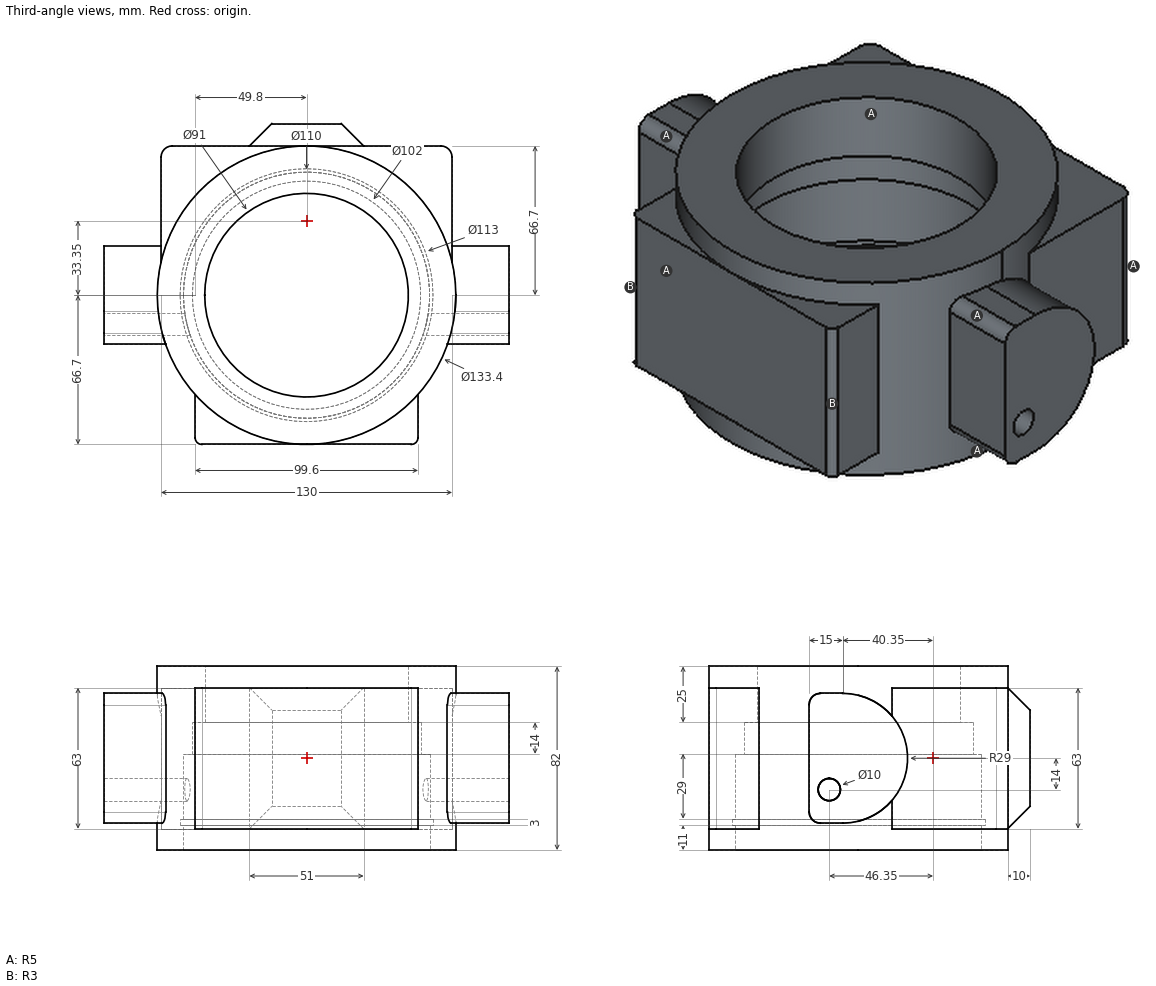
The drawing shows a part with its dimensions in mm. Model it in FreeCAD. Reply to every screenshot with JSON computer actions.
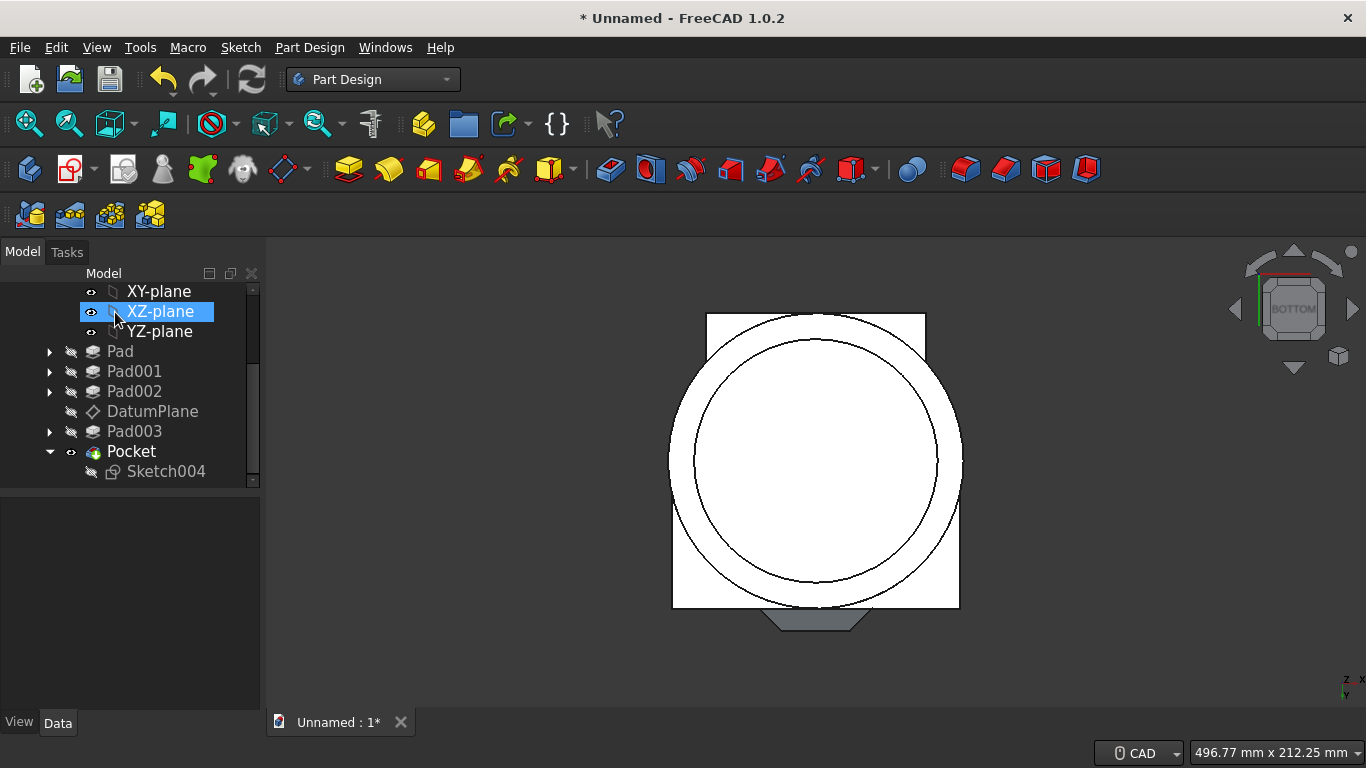
{"action": "left_click", "coordinate": [816, 460]}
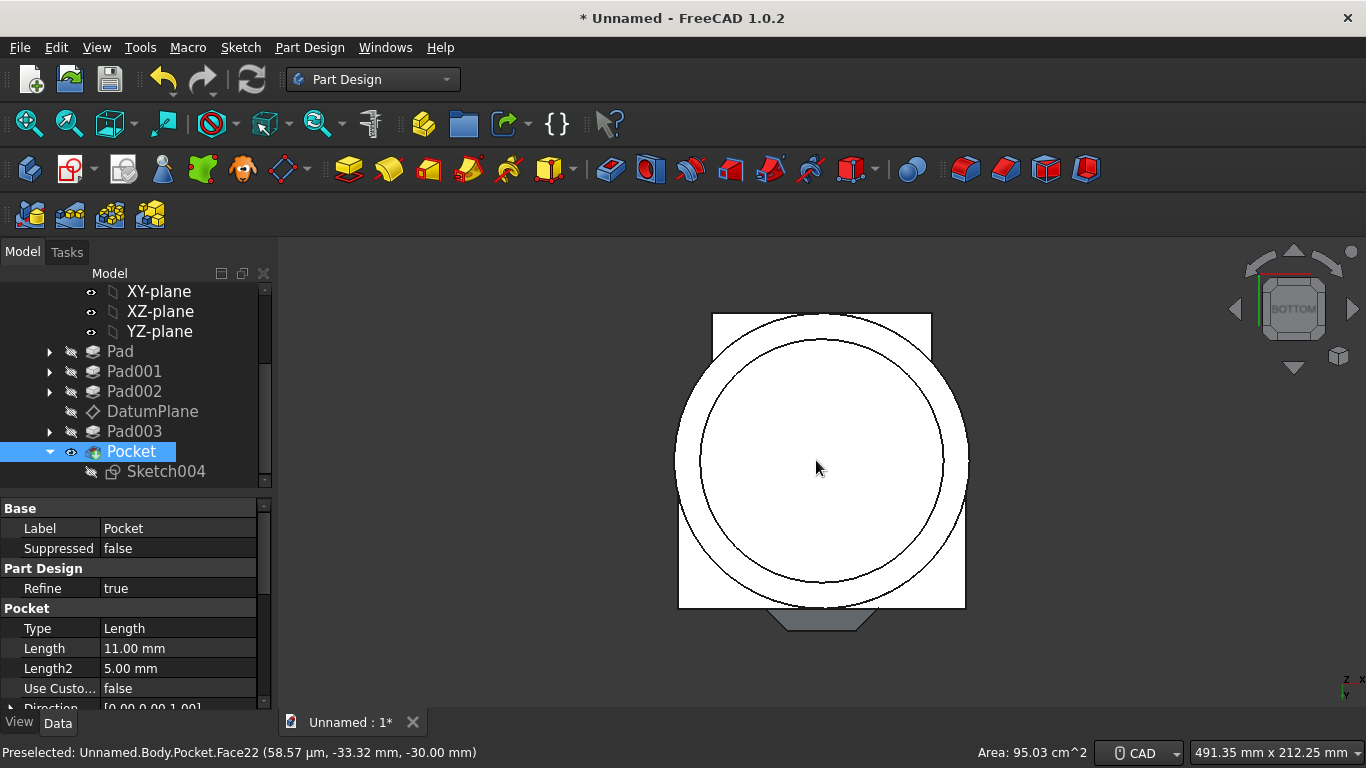
{"action": "left_click", "coordinate": [70, 170]}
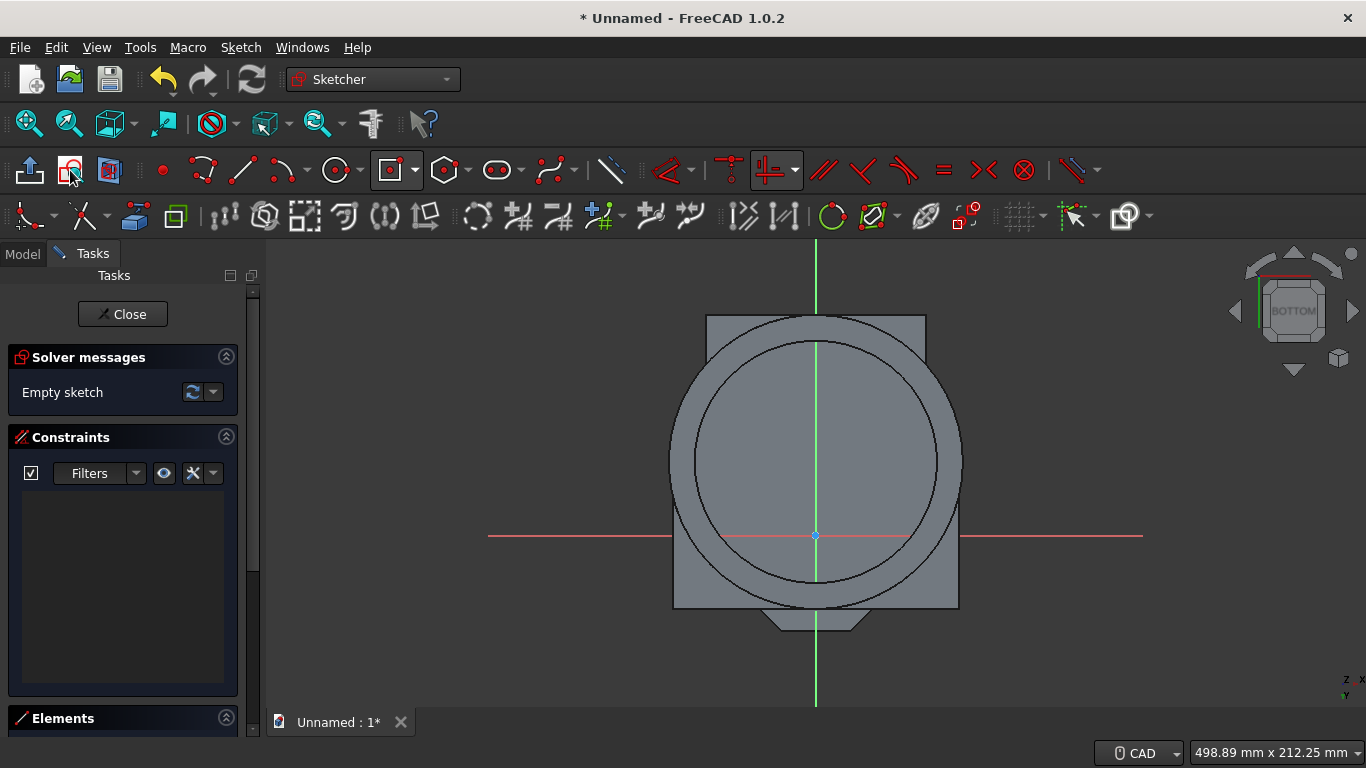
{"action": "key", "text": "q s"}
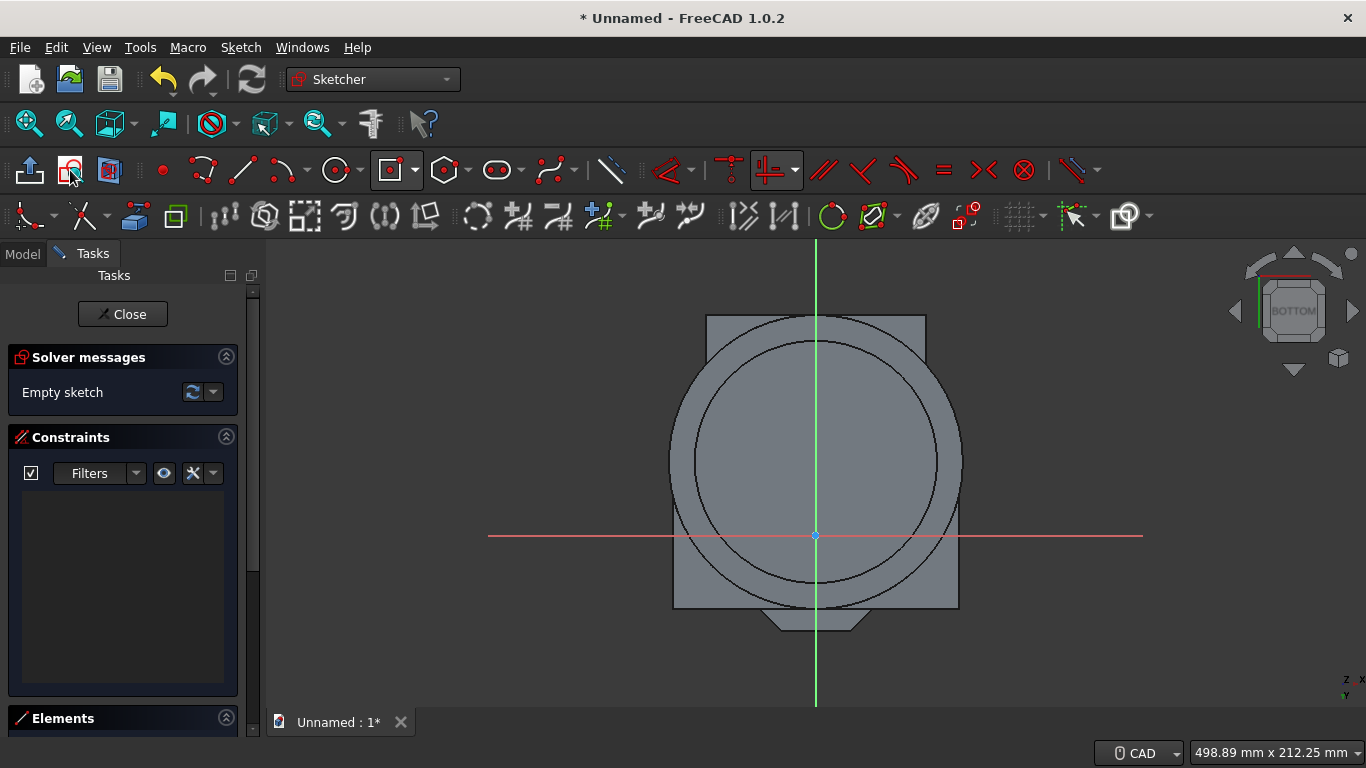
{"action": "key", "text": "g c"}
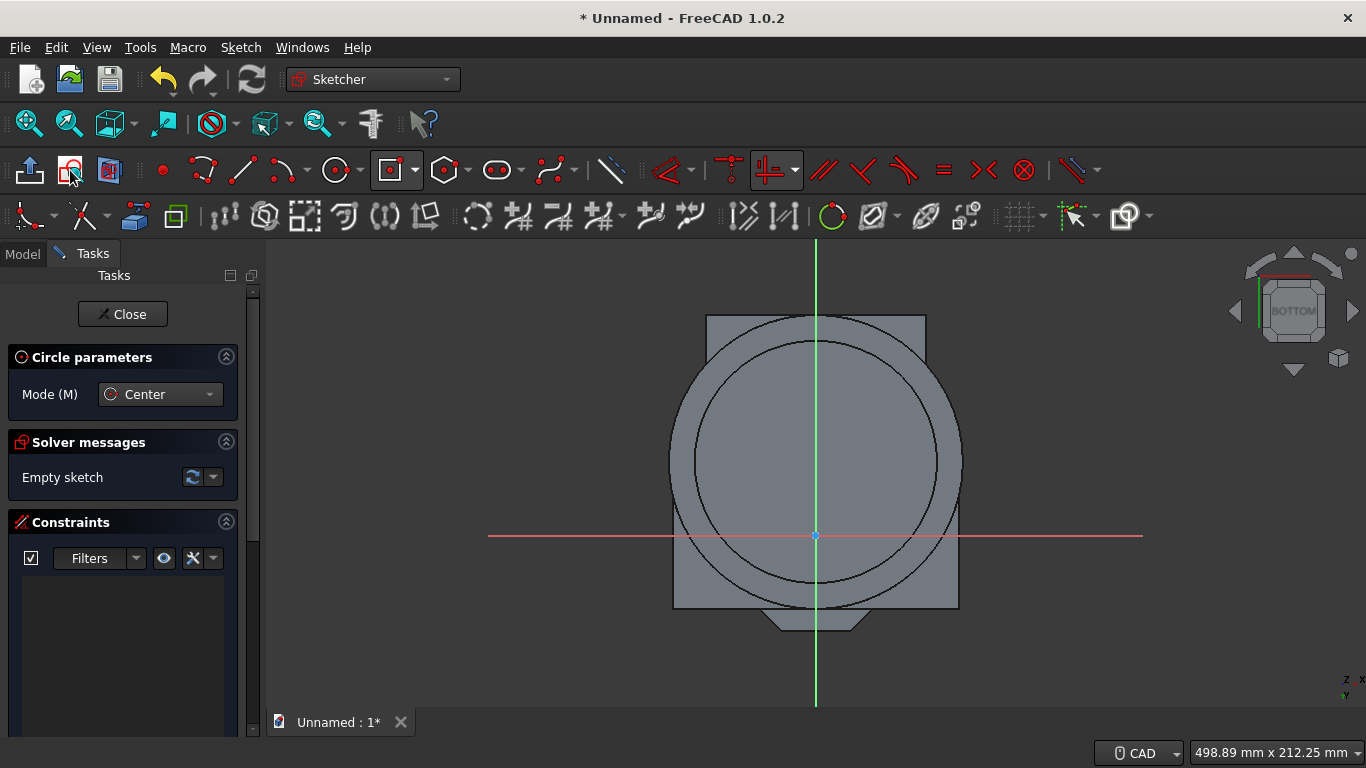
{"action": "left_click", "coordinate": [816, 462]}
{"action": "left_click", "coordinate": [904, 374]}
{"action": "key", "text": "Escape"}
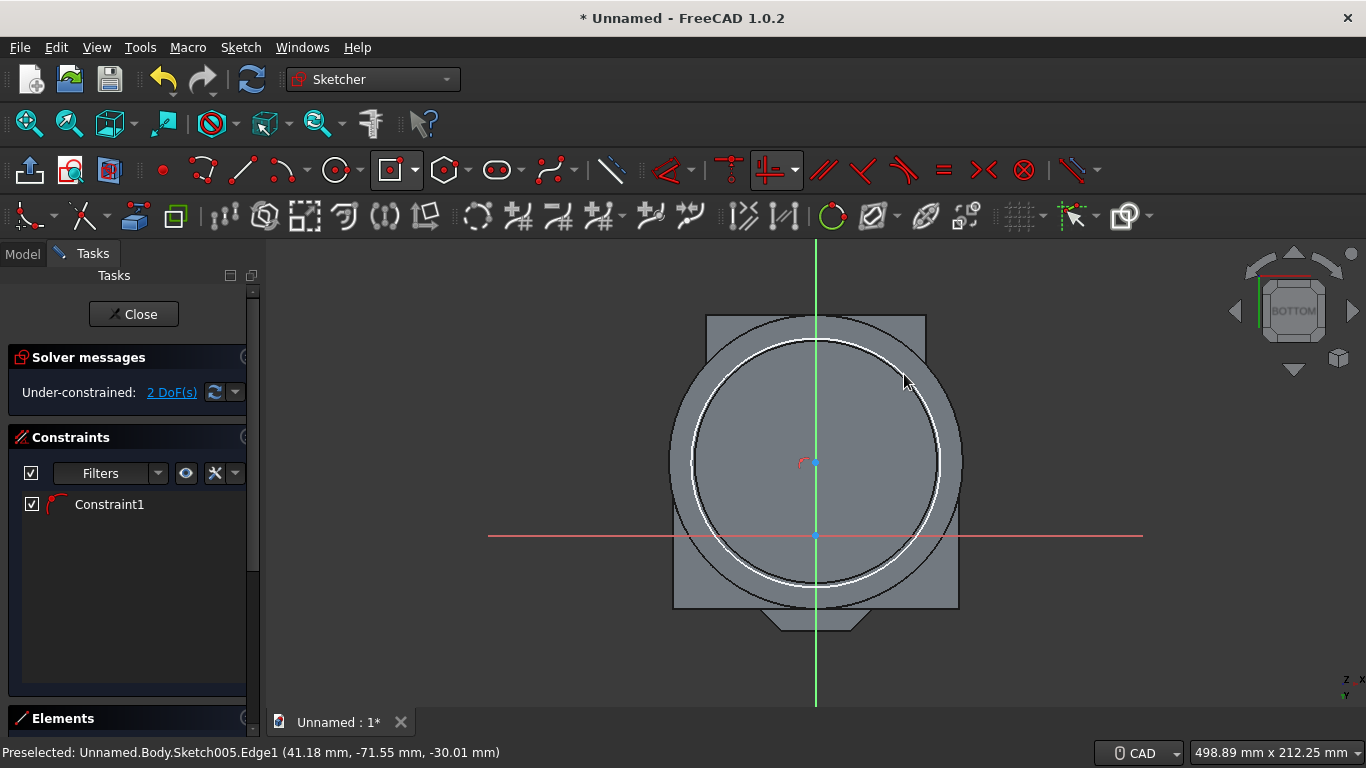
{"action": "key", "text": "d"}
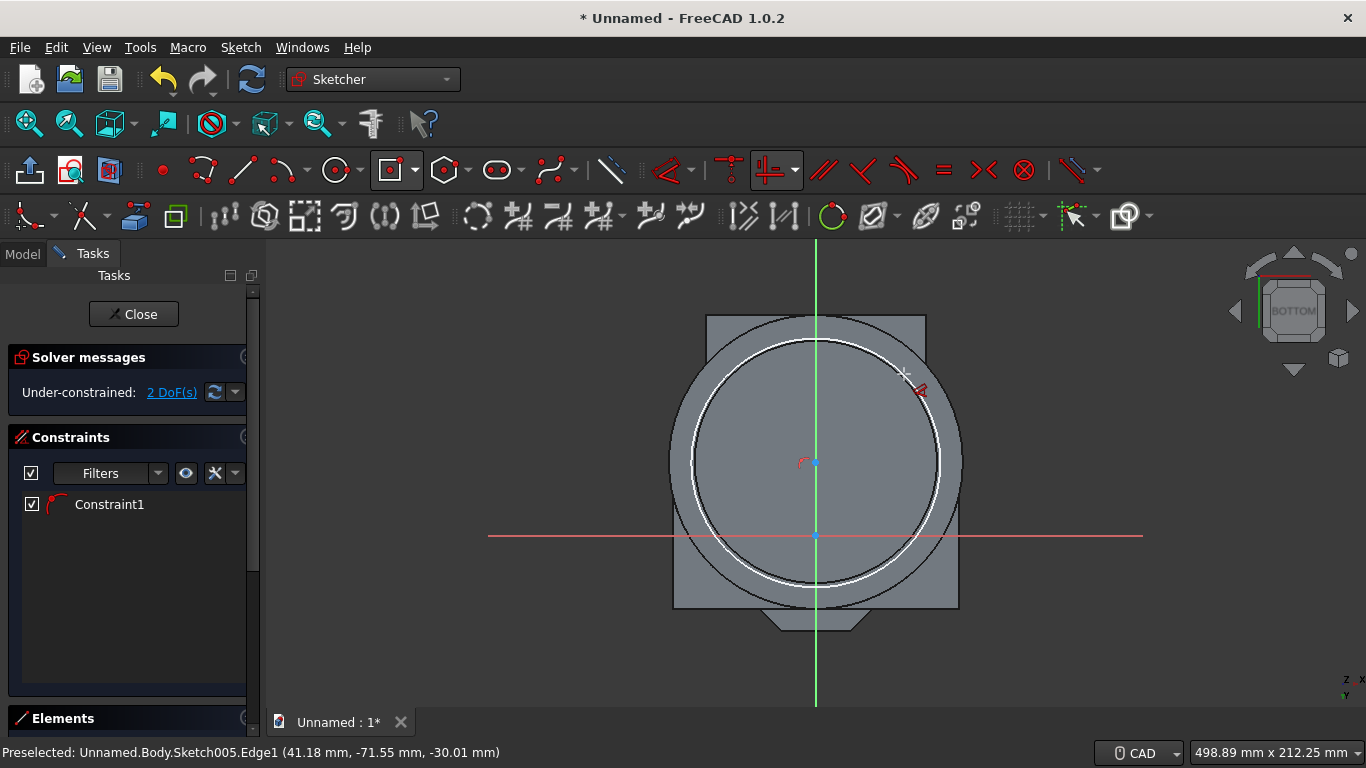
{"action": "left_click", "coordinate": [904, 375]}
{"action": "left_click", "coordinate": [927, 352]}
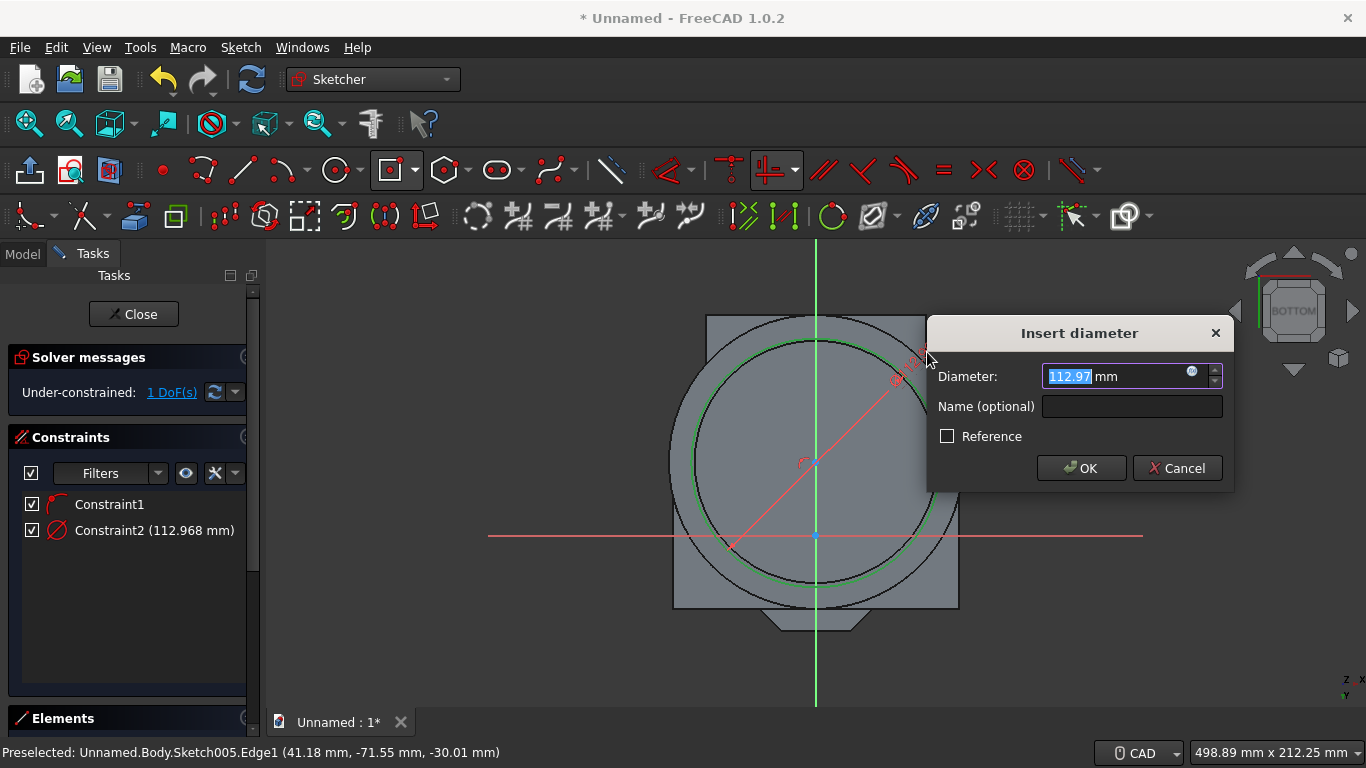
{"action": "type", "text": "113"}
{"action": "key", "text": "Return"}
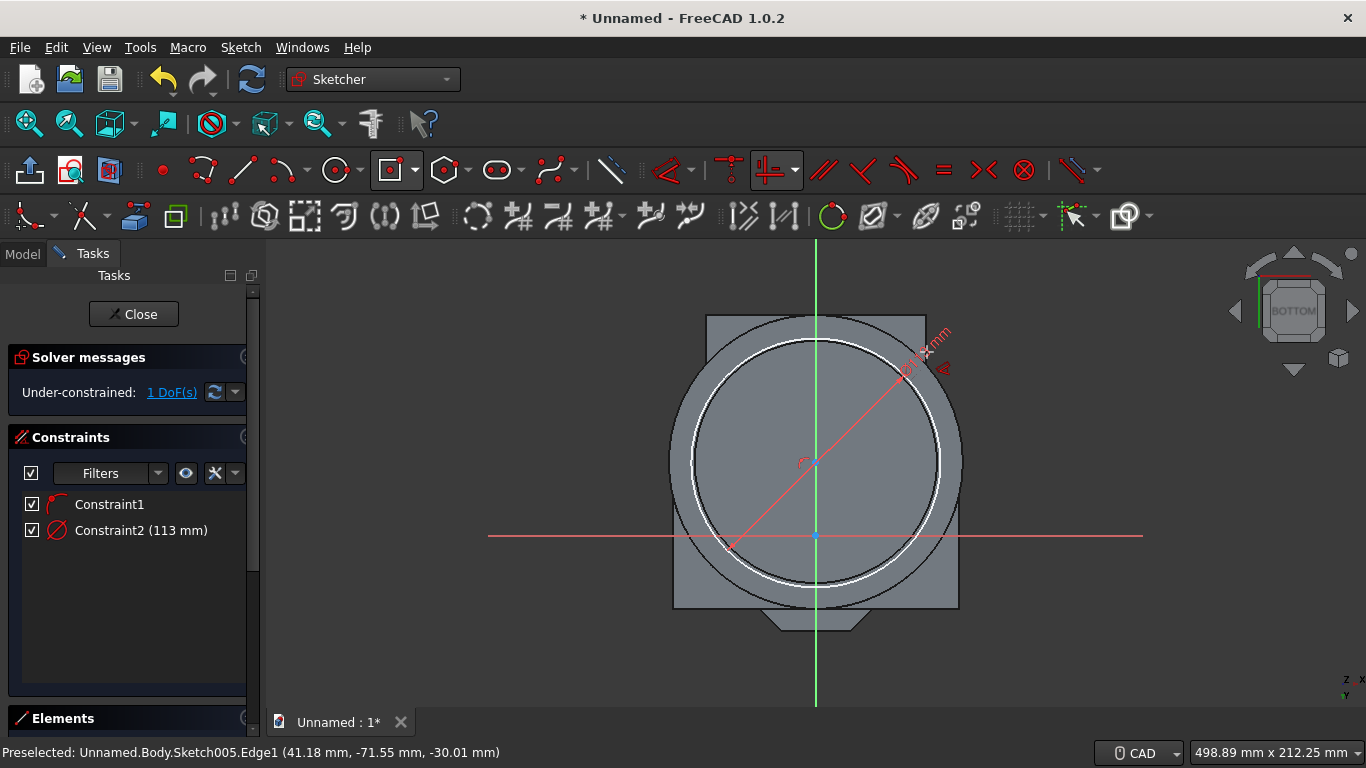
{"action": "left_click", "coordinate": [816, 463]}
{"action": "left_click", "coordinate": [850, 499]}